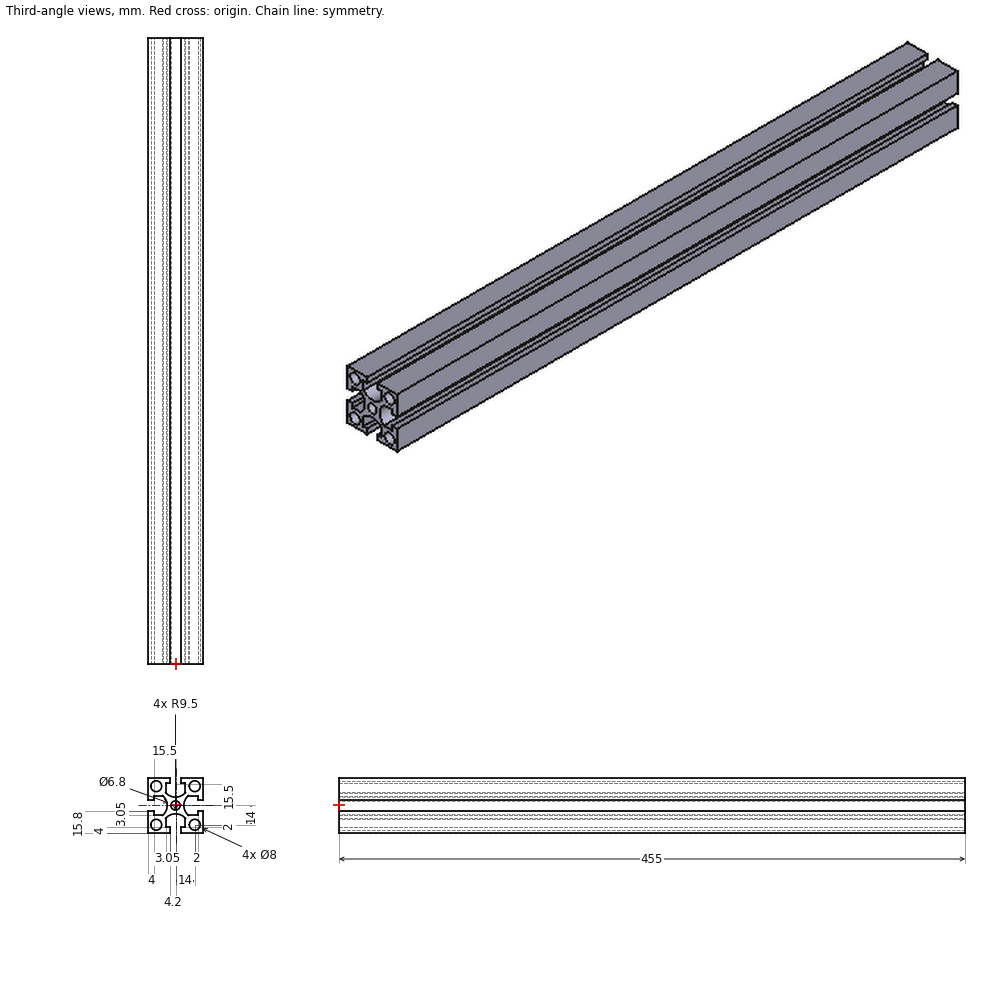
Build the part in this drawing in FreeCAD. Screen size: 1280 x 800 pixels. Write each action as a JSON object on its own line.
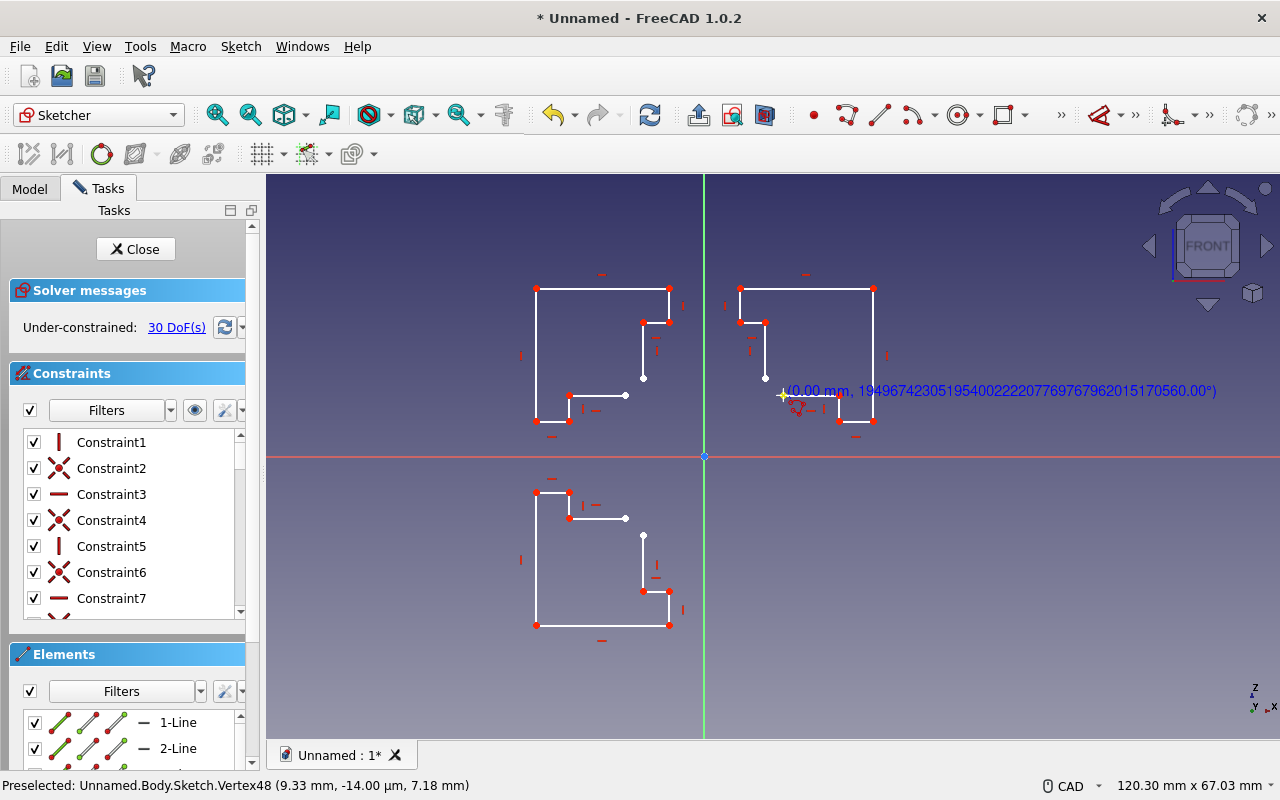
{"action": "left_click", "coordinate": [783, 518]}
{"action": "left_click", "coordinate": [839, 518]}
{"action": "left_click", "coordinate": [839, 492]}
{"action": "left_click", "coordinate": [873, 492]}
{"action": "left_click", "coordinate": [873, 625]}
{"action": "left_click", "coordinate": [740, 625]}
{"action": "left_click", "coordinate": [740, 591]}
{"action": "left_click", "coordinate": [765, 591]}
{"action": "left_click", "coordinate": [765, 535]}
{"action": "right_click", "coordinate": [765, 535]}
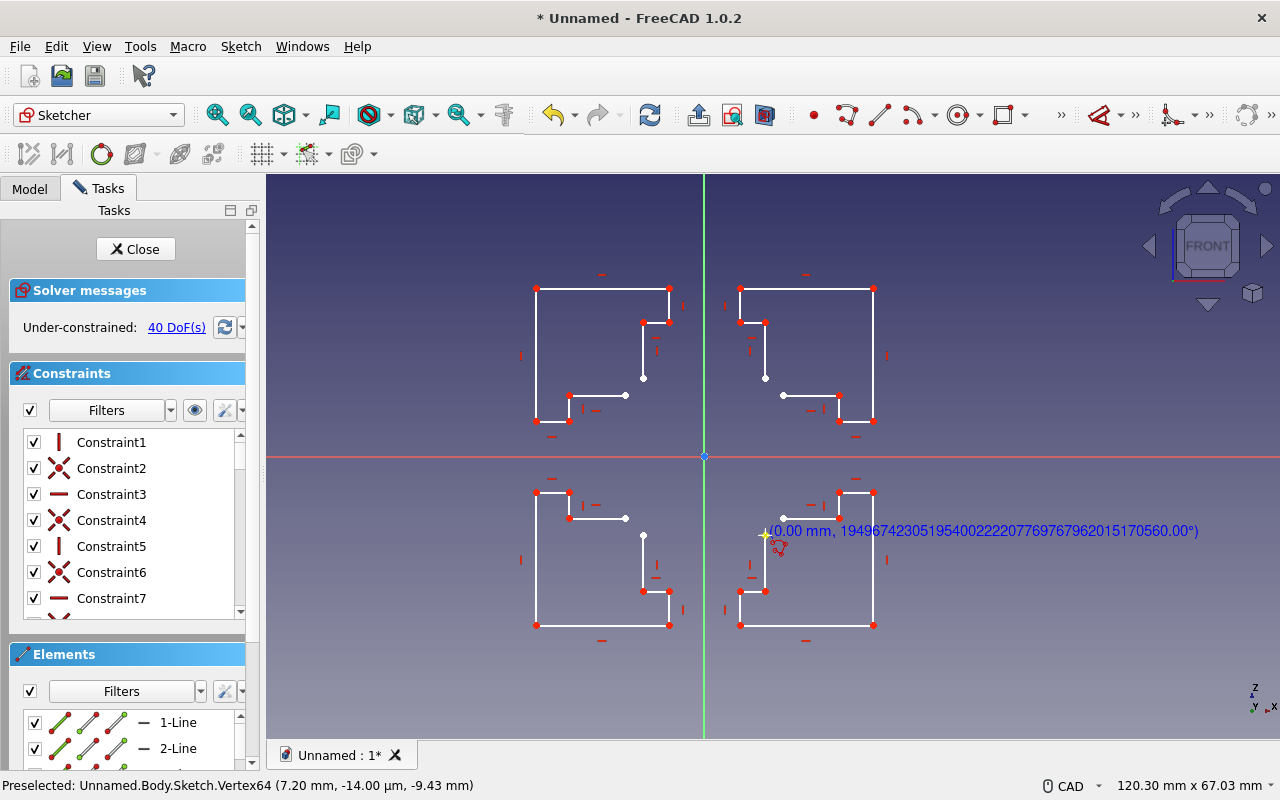
{"action": "left_click", "coordinate": [934, 116]}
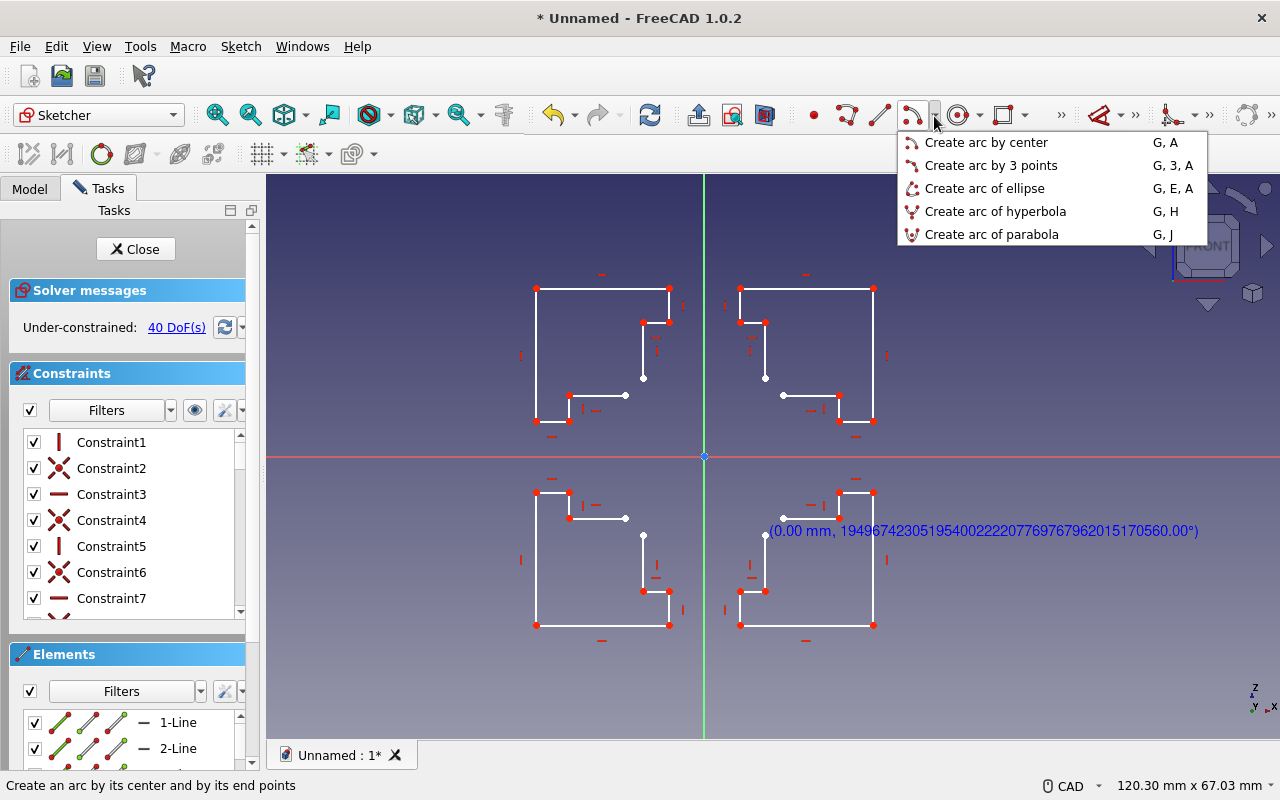
{"action": "left_click", "coordinate": [1052, 166]}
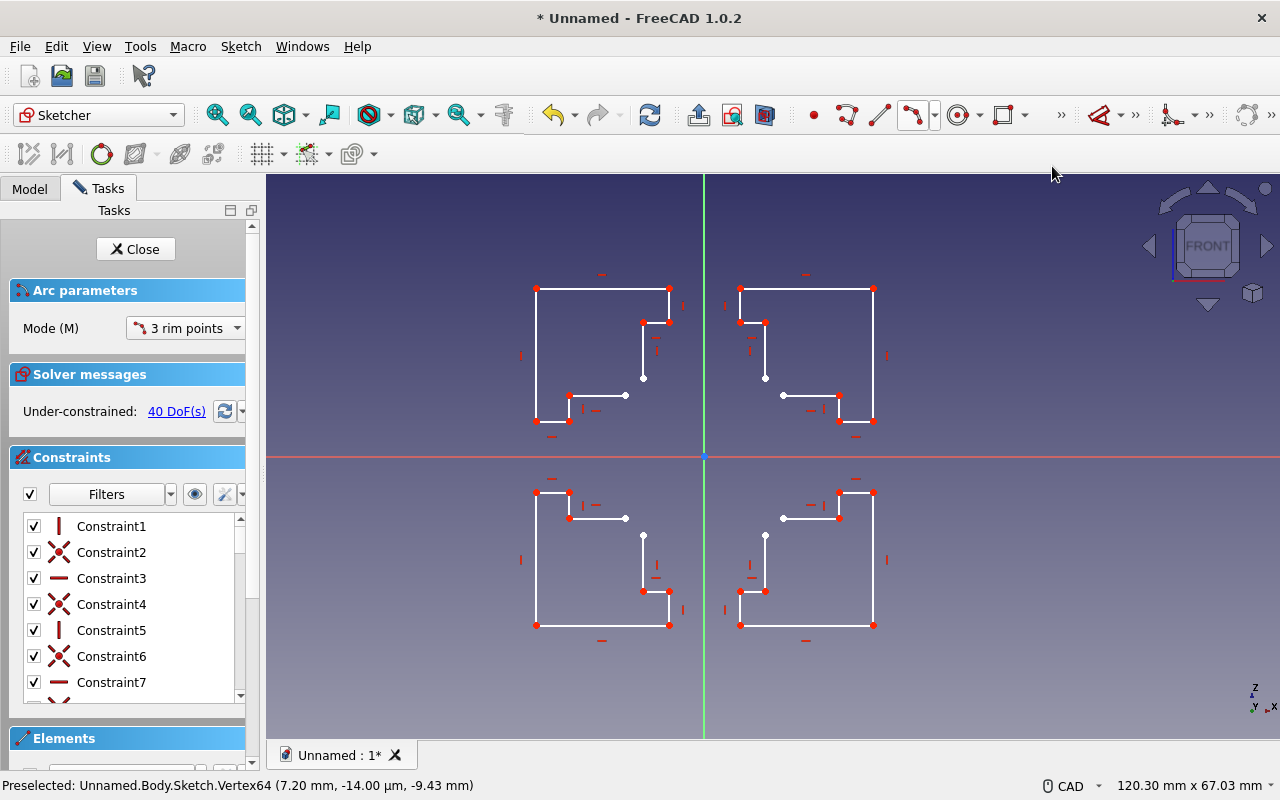
{"action": "left_click", "coordinate": [625, 519]}
{"action": "left_click", "coordinate": [625, 396]}
{"action": "left_click", "coordinate": [649, 484]}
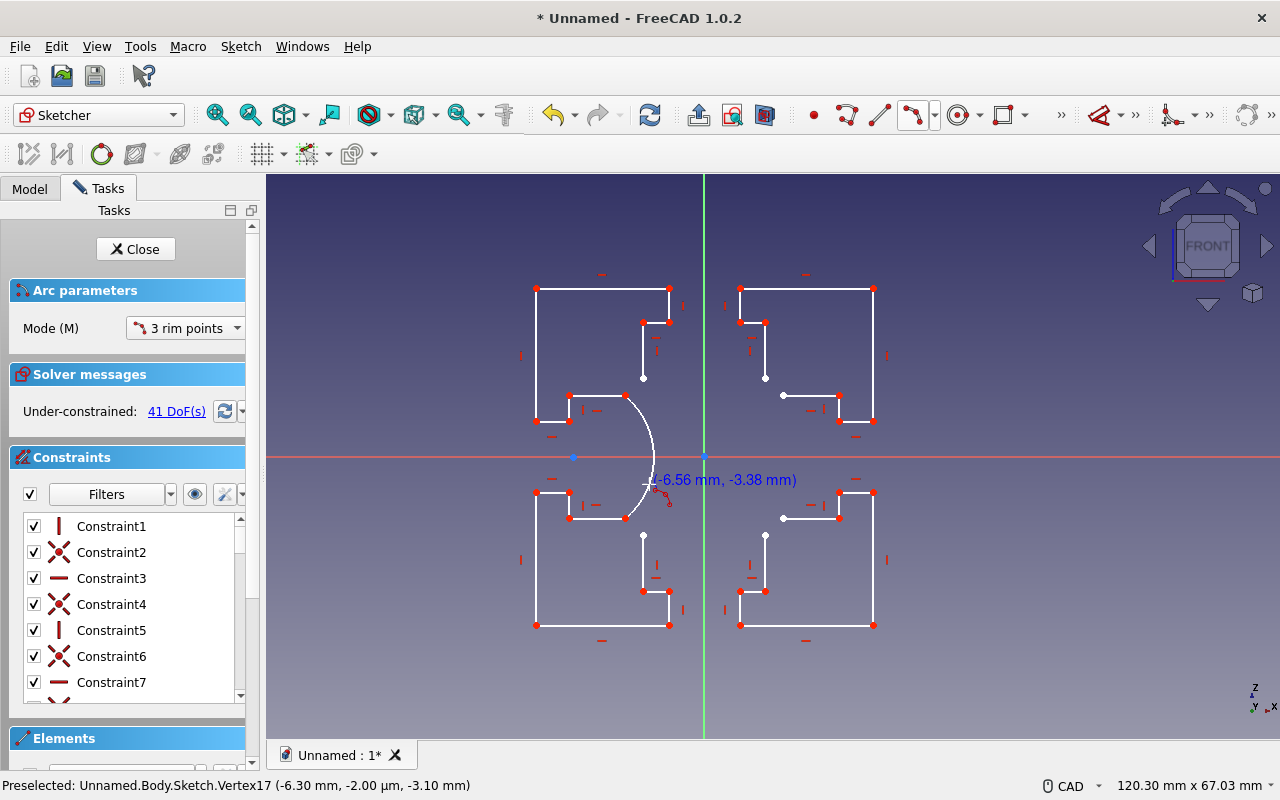
{"action": "left_click", "coordinate": [643, 379]}
{"action": "left_click", "coordinate": [765, 379]}
{"action": "left_click", "coordinate": [677, 401]}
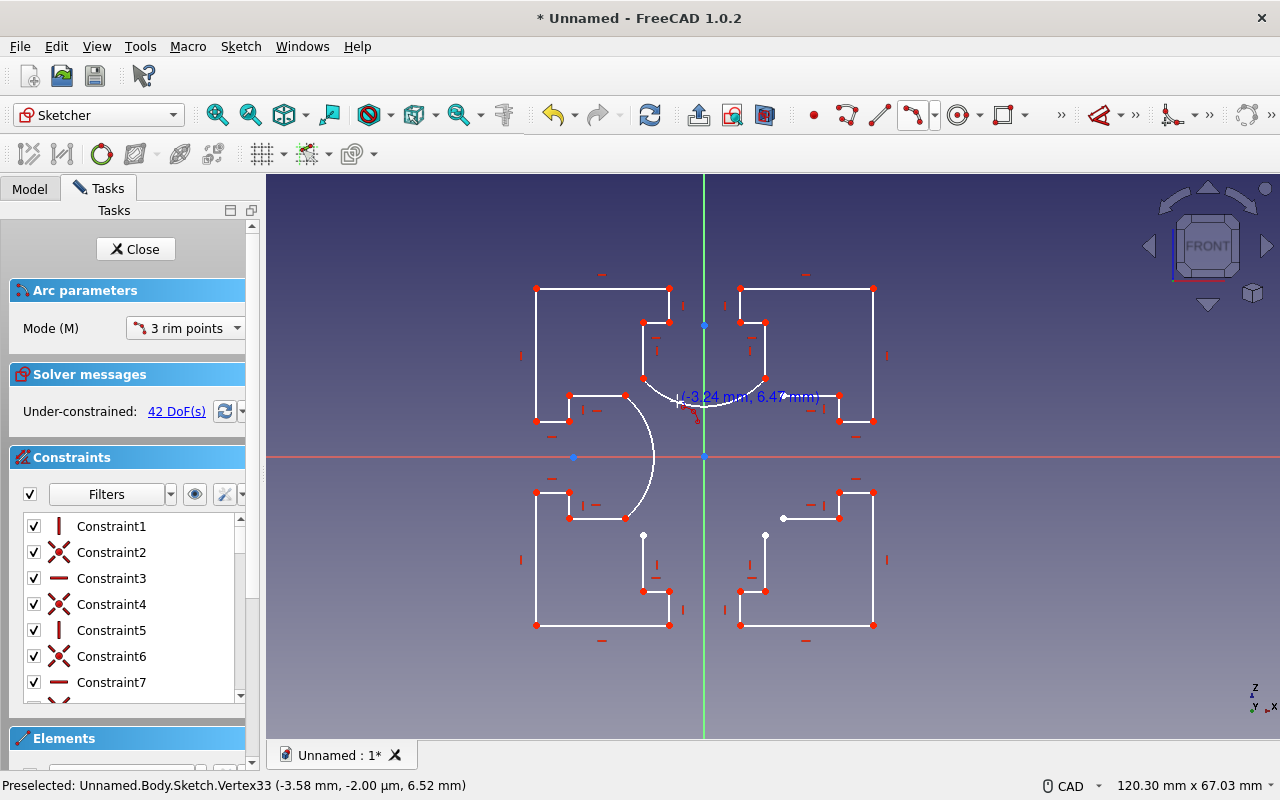
{"action": "left_click", "coordinate": [783, 396]}
{"action": "left_click", "coordinate": [783, 519]}
{"action": "left_click", "coordinate": [760, 429]}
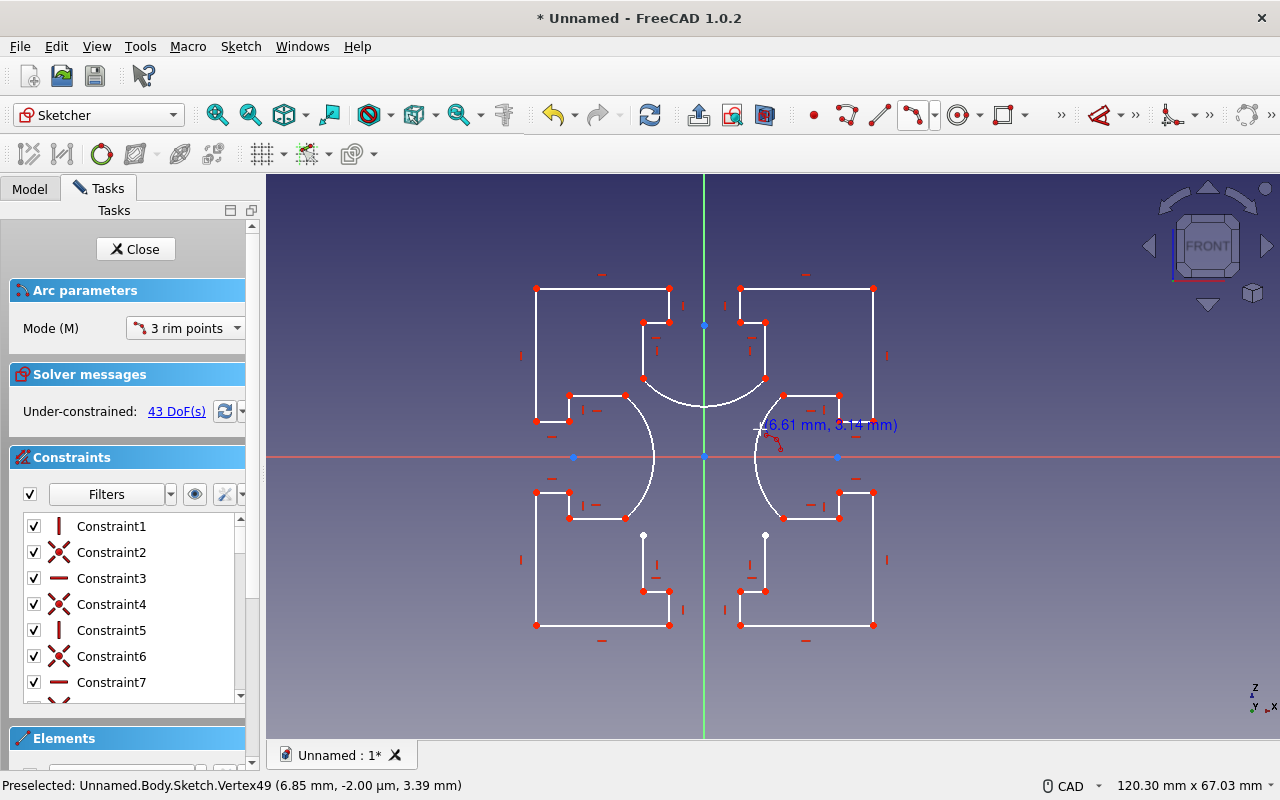
{"action": "left_click", "coordinate": [765, 536]}
{"action": "left_click", "coordinate": [643, 536]}
{"action": "left_click", "coordinate": [732, 512]}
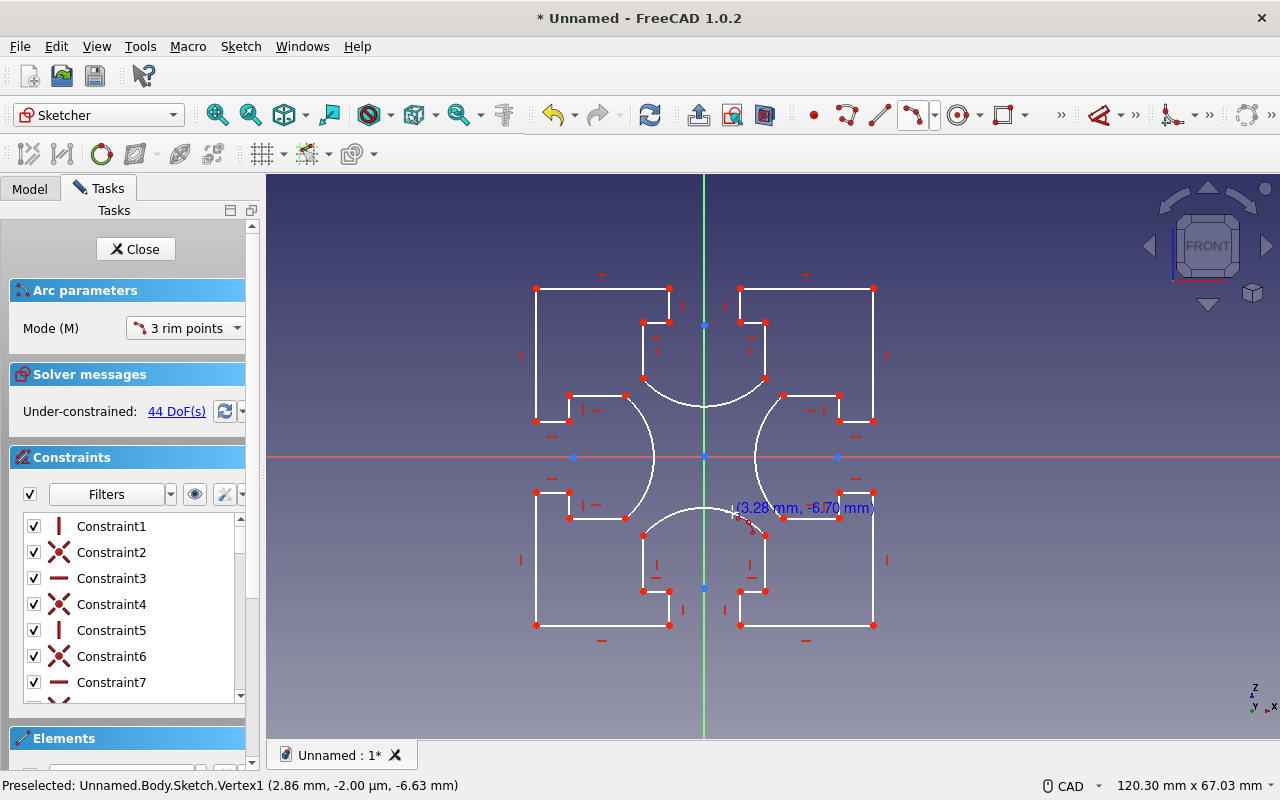
{"action": "left_click", "coordinate": [958, 116]}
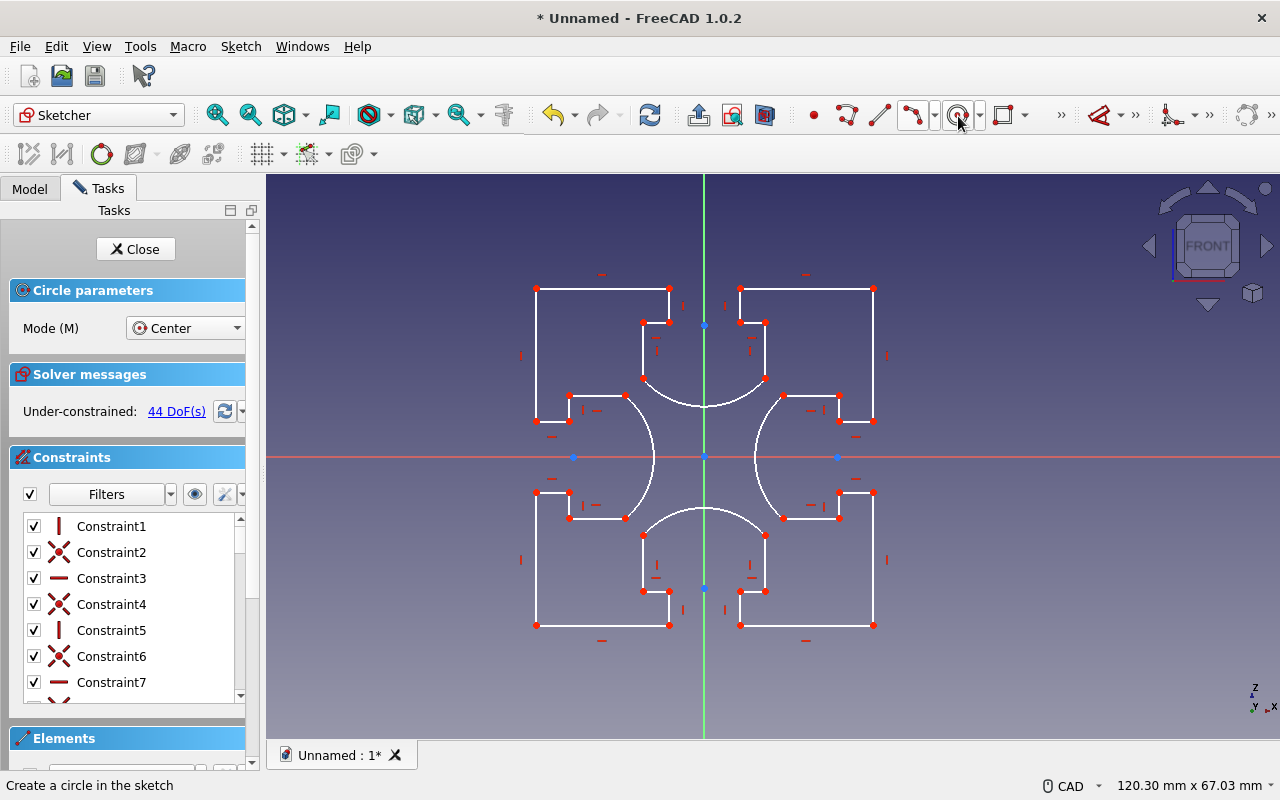
{"action": "left_click", "coordinate": [822, 575]}
{"action": "left_click", "coordinate": [846, 551]}